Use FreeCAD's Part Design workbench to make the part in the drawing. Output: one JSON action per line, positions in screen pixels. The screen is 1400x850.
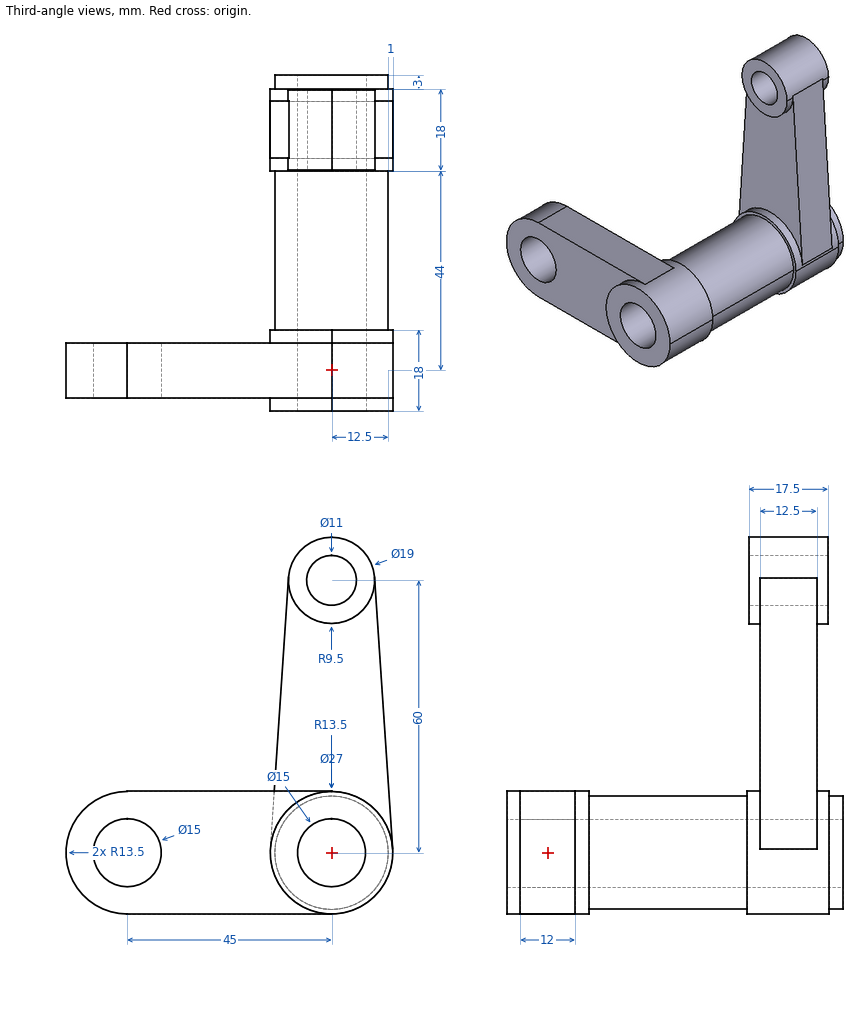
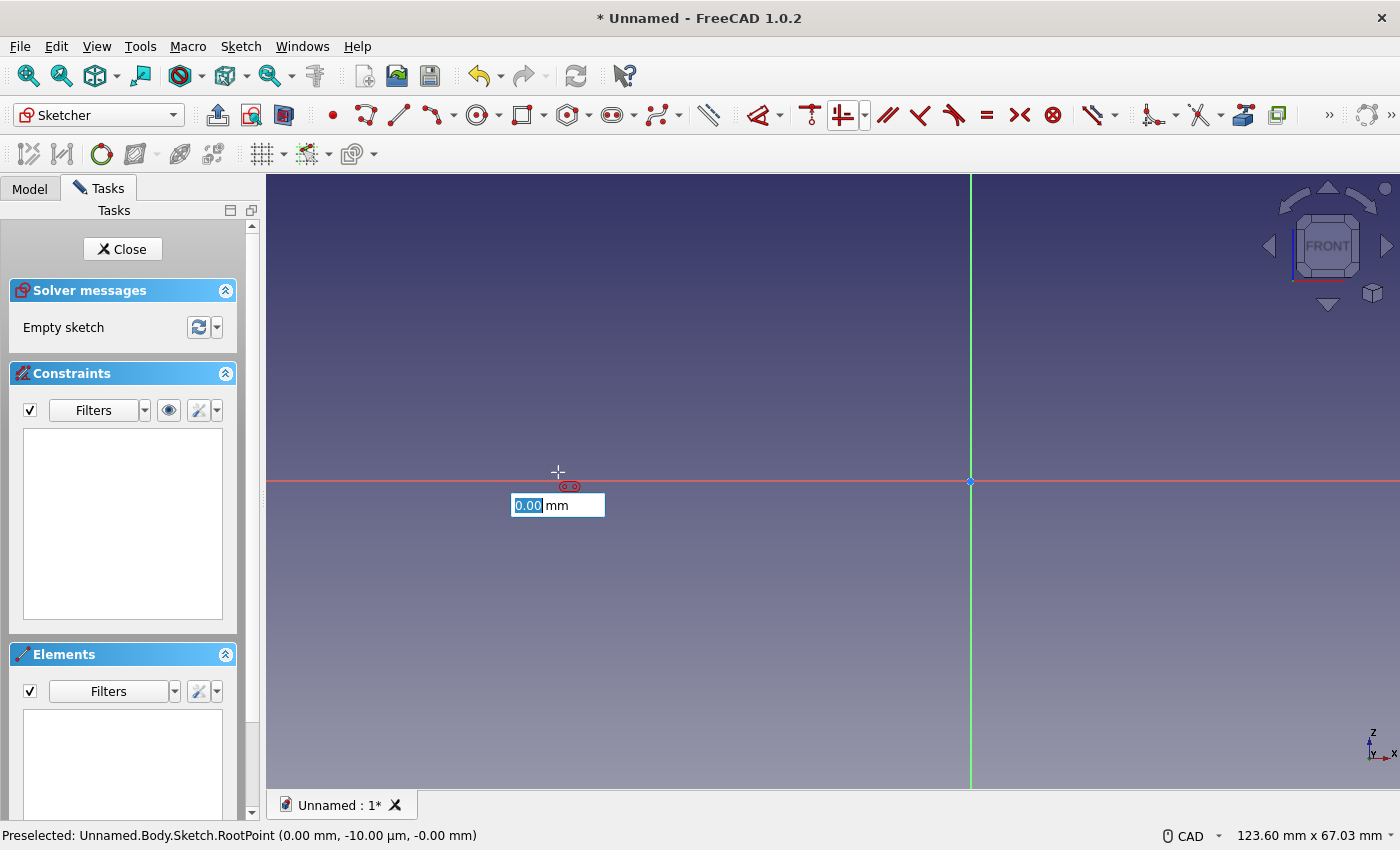
{"action": "left_click", "coordinate": [764, 605]}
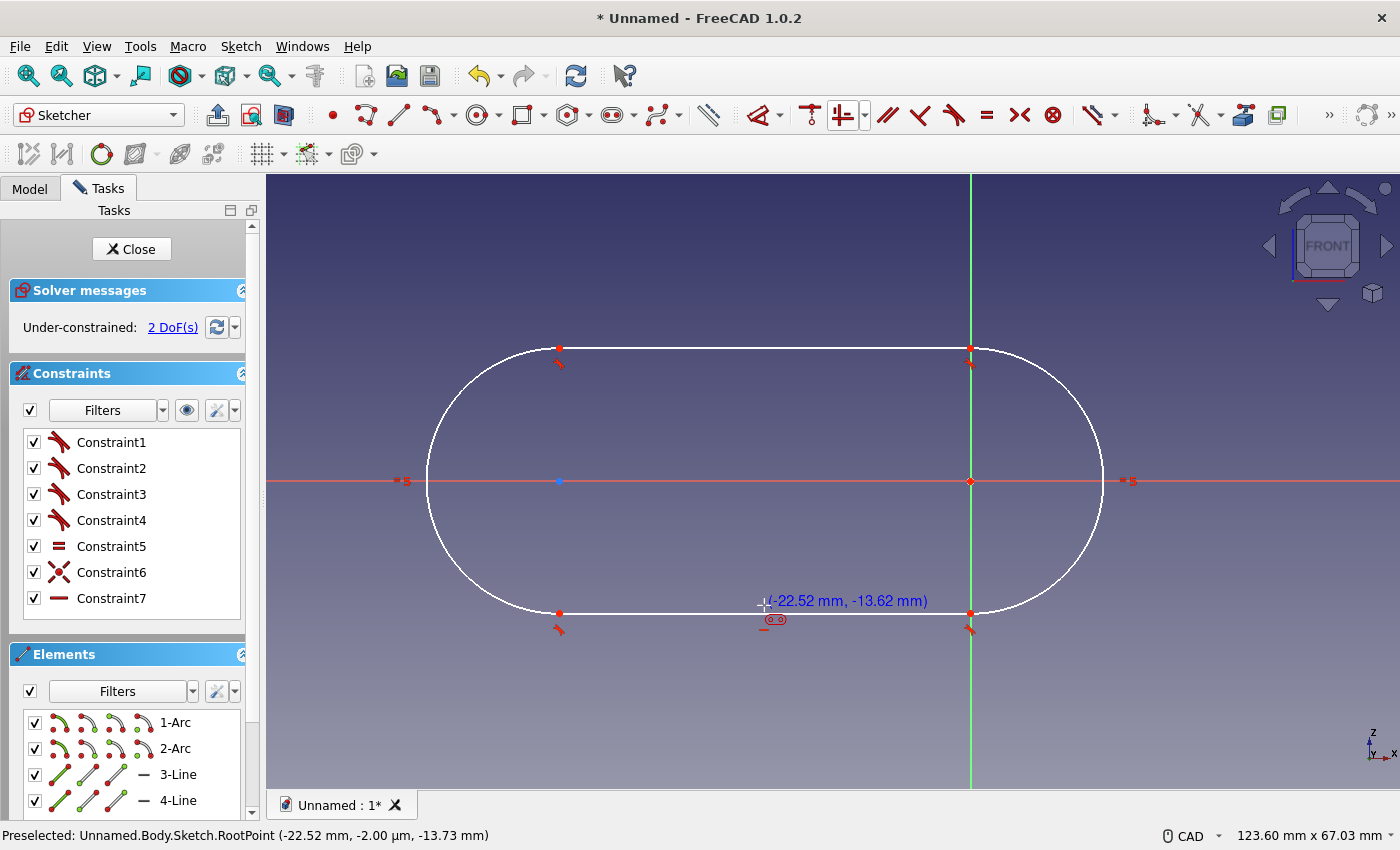
{"action": "left_click", "coordinate": [476, 116]}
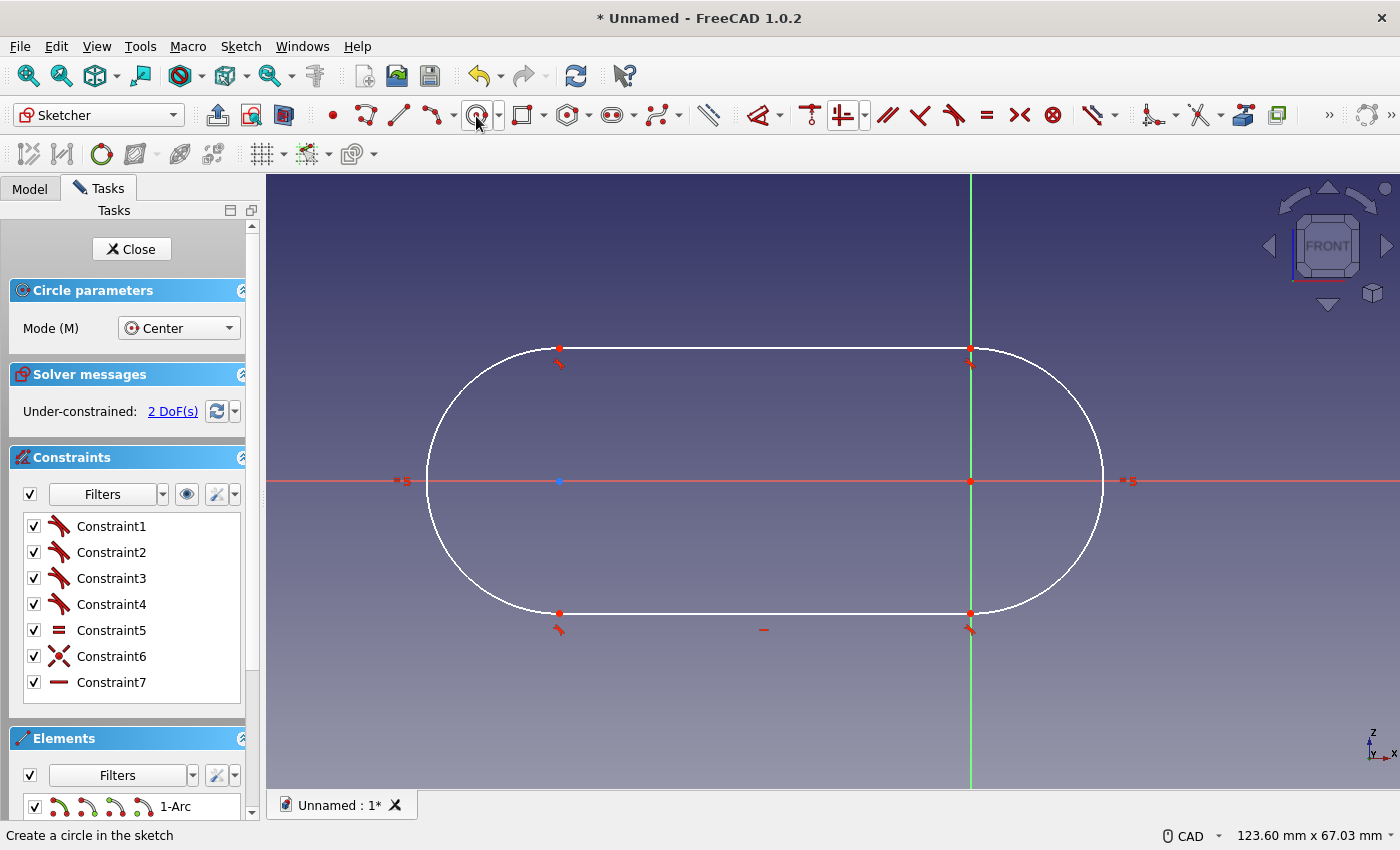
{"action": "left_click", "coordinate": [558, 472]}
{"action": "left_click", "coordinate": [606, 432]}
{"action": "key", "text": "Escape"}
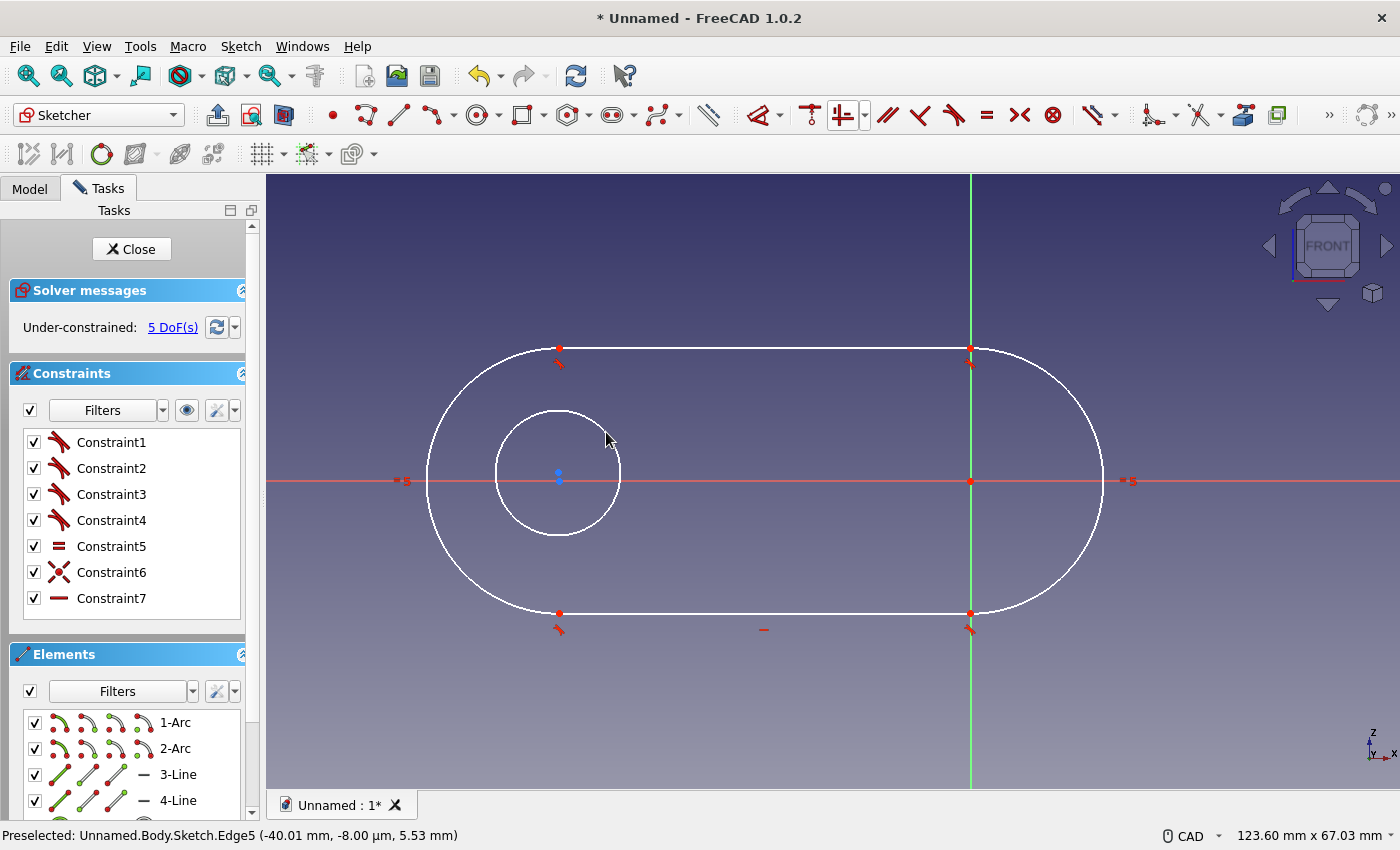
{"action": "left_click", "coordinate": [602, 429]}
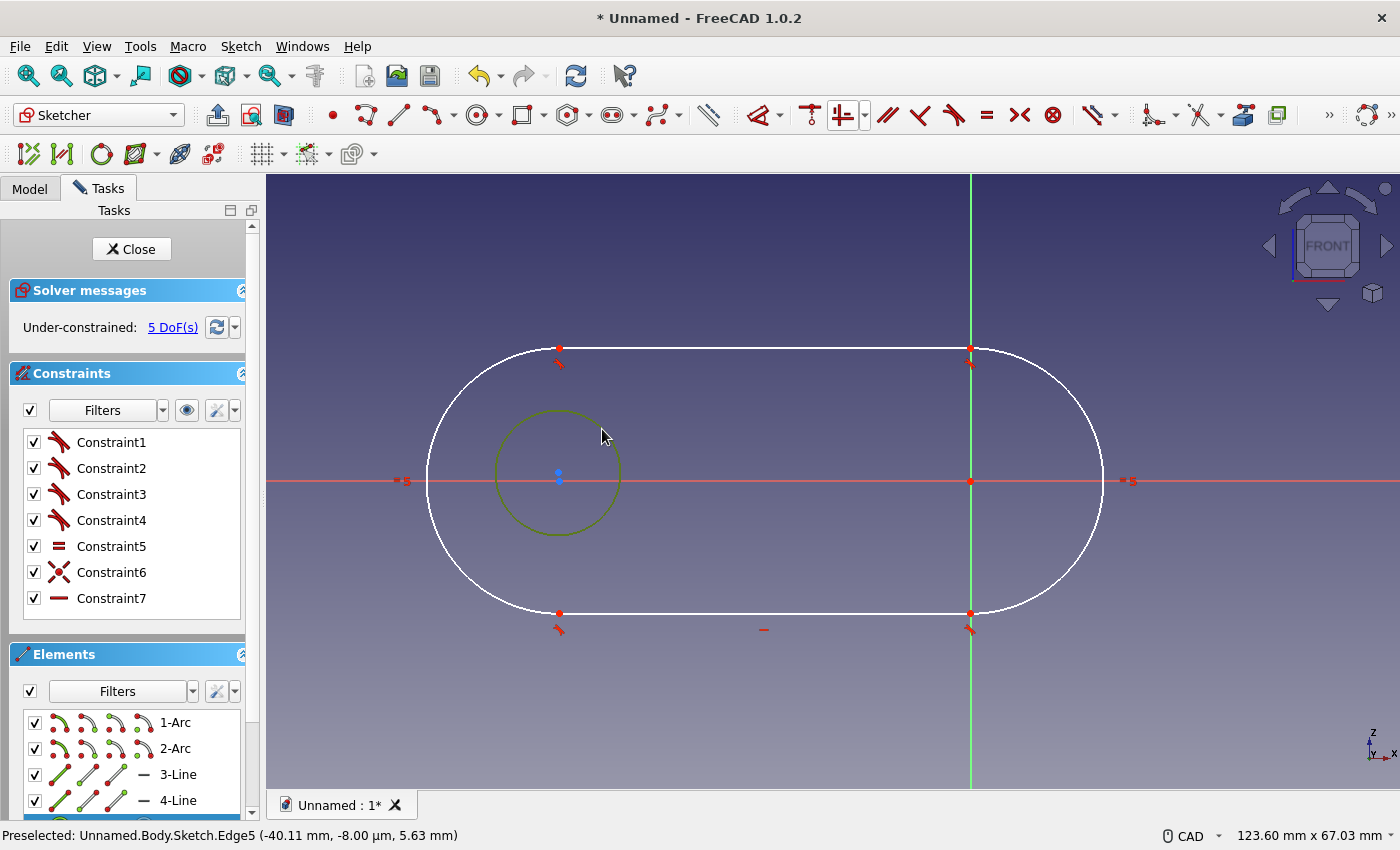
{"action": "left_click", "coordinate": [452, 403]}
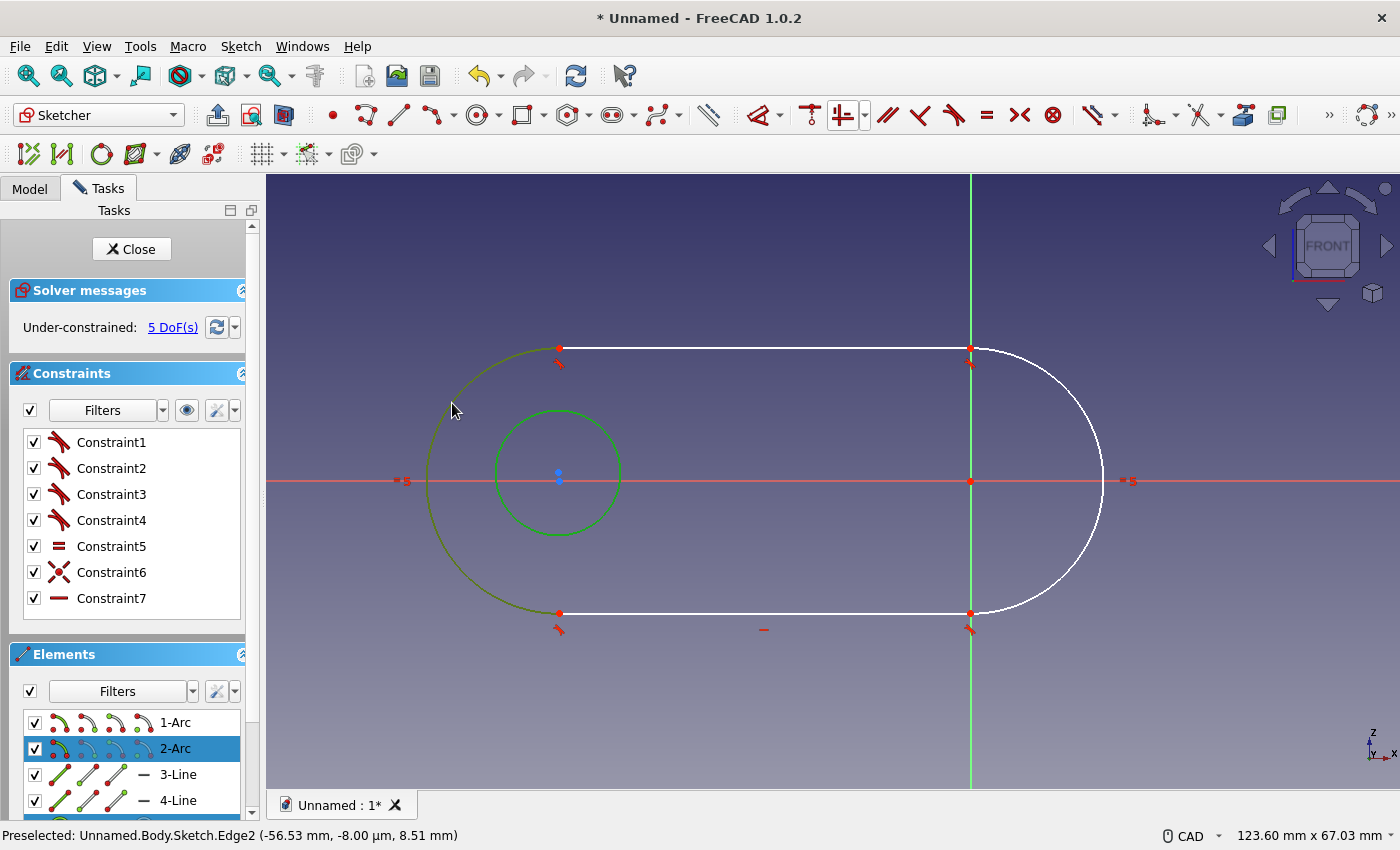
{"action": "key", "text": "c"}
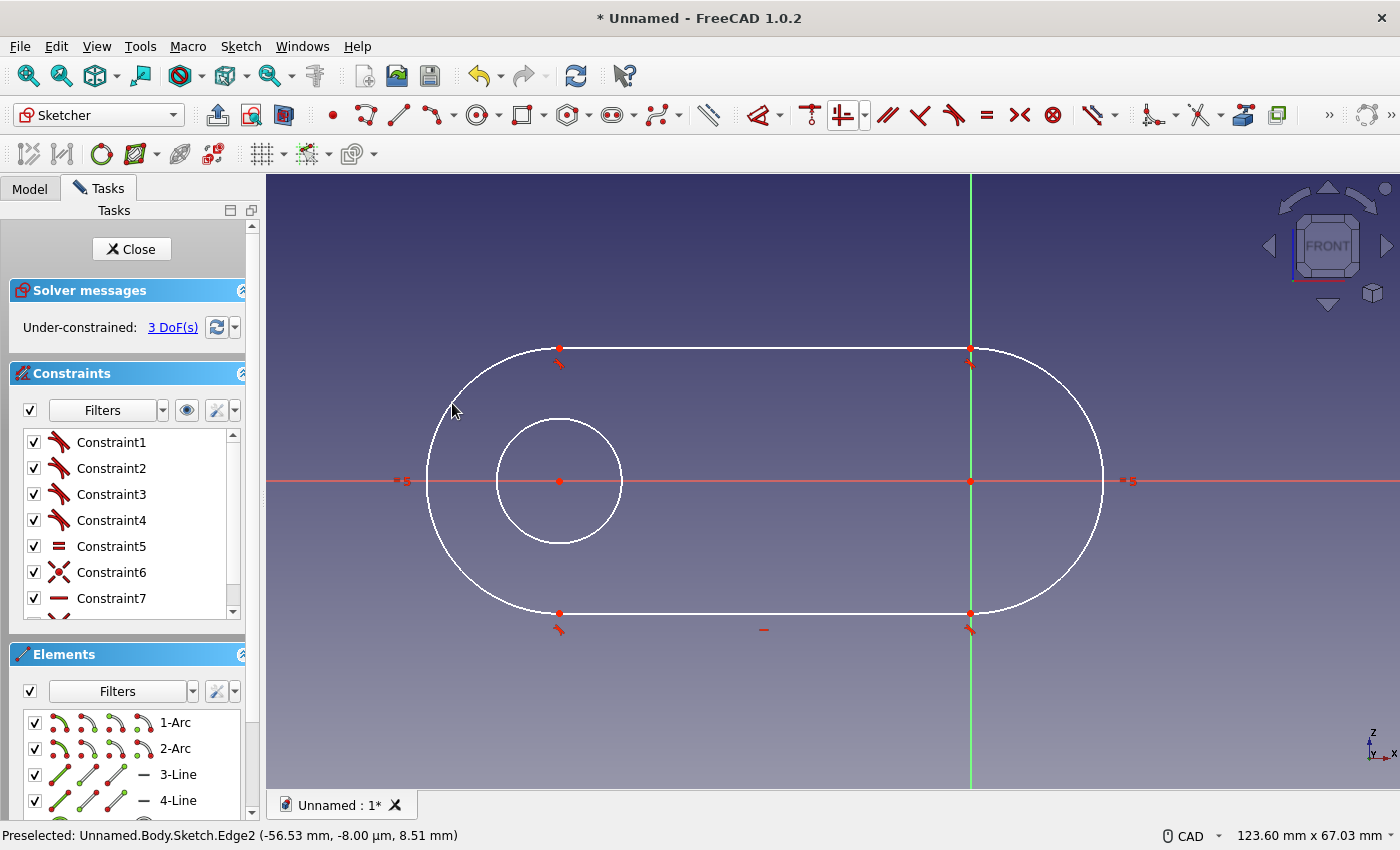
{"action": "key", "text": "d"}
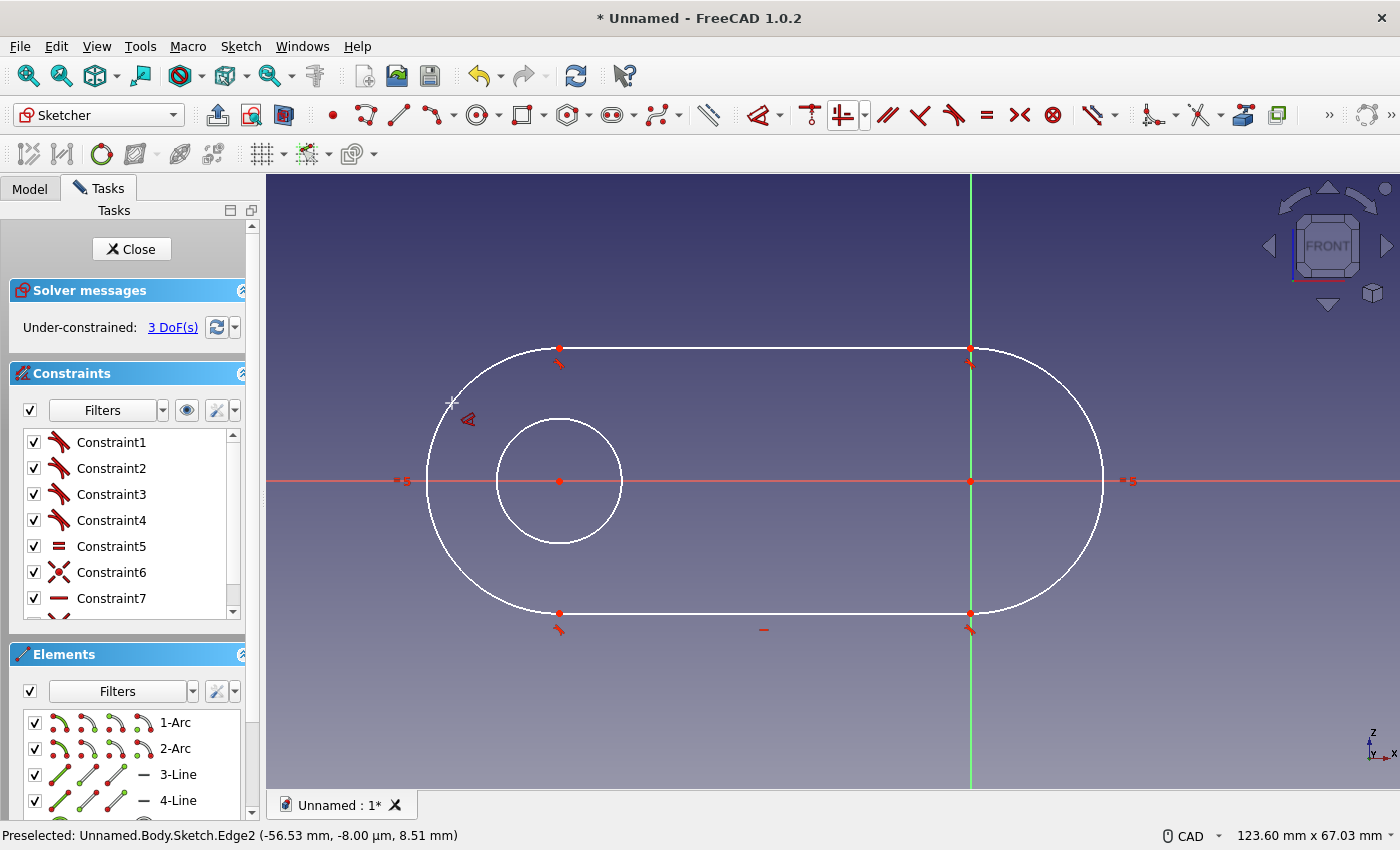
{"action": "left_click", "coordinate": [1078, 559]}
{"action": "left_click", "coordinate": [1104, 578]}